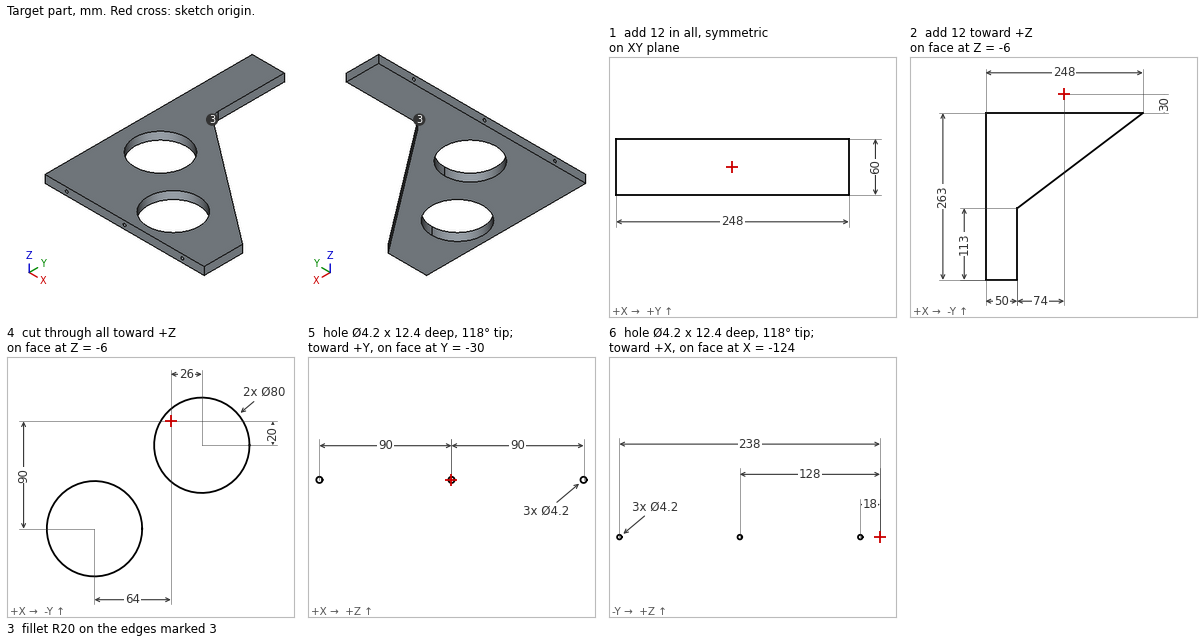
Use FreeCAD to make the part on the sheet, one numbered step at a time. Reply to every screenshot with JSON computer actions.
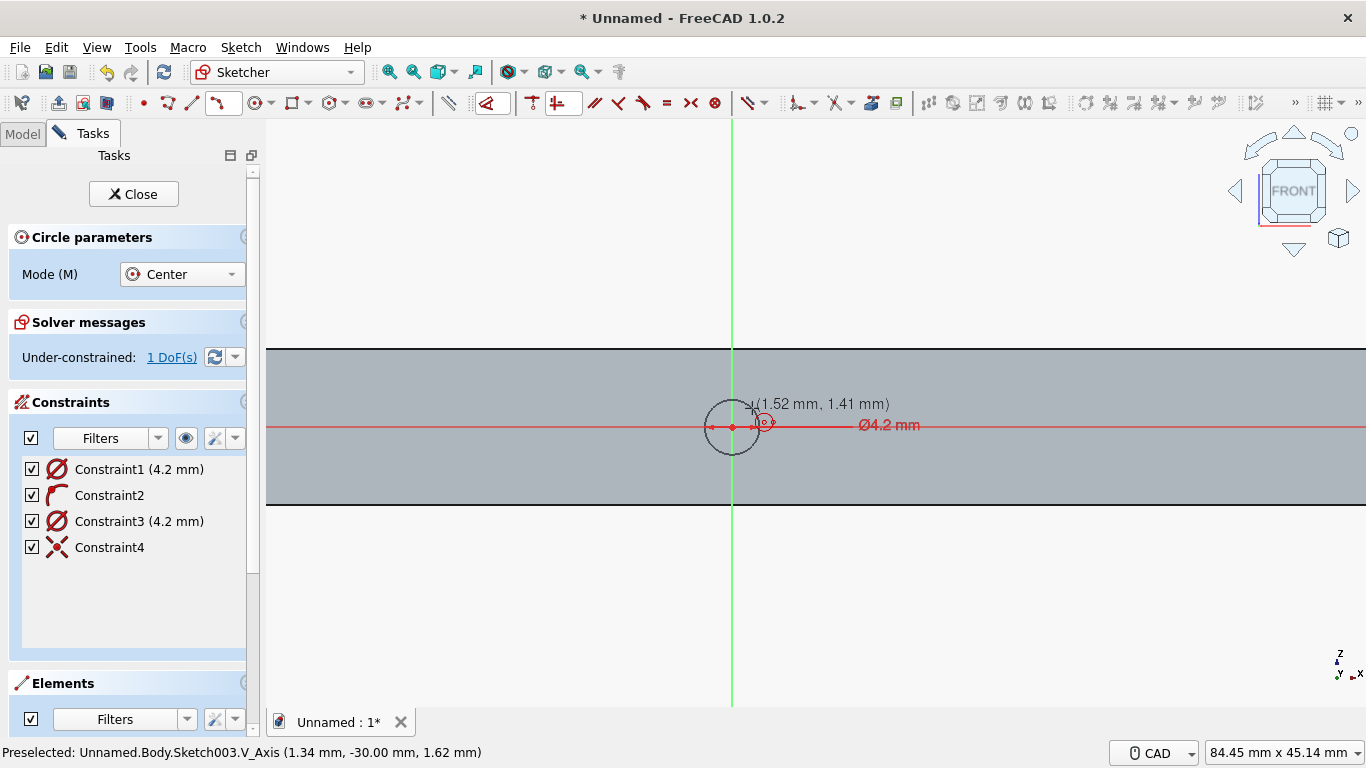
{"action": "scroll", "coordinate": [753, 408], "scroll_direction": "down", "scroll_amount": 7}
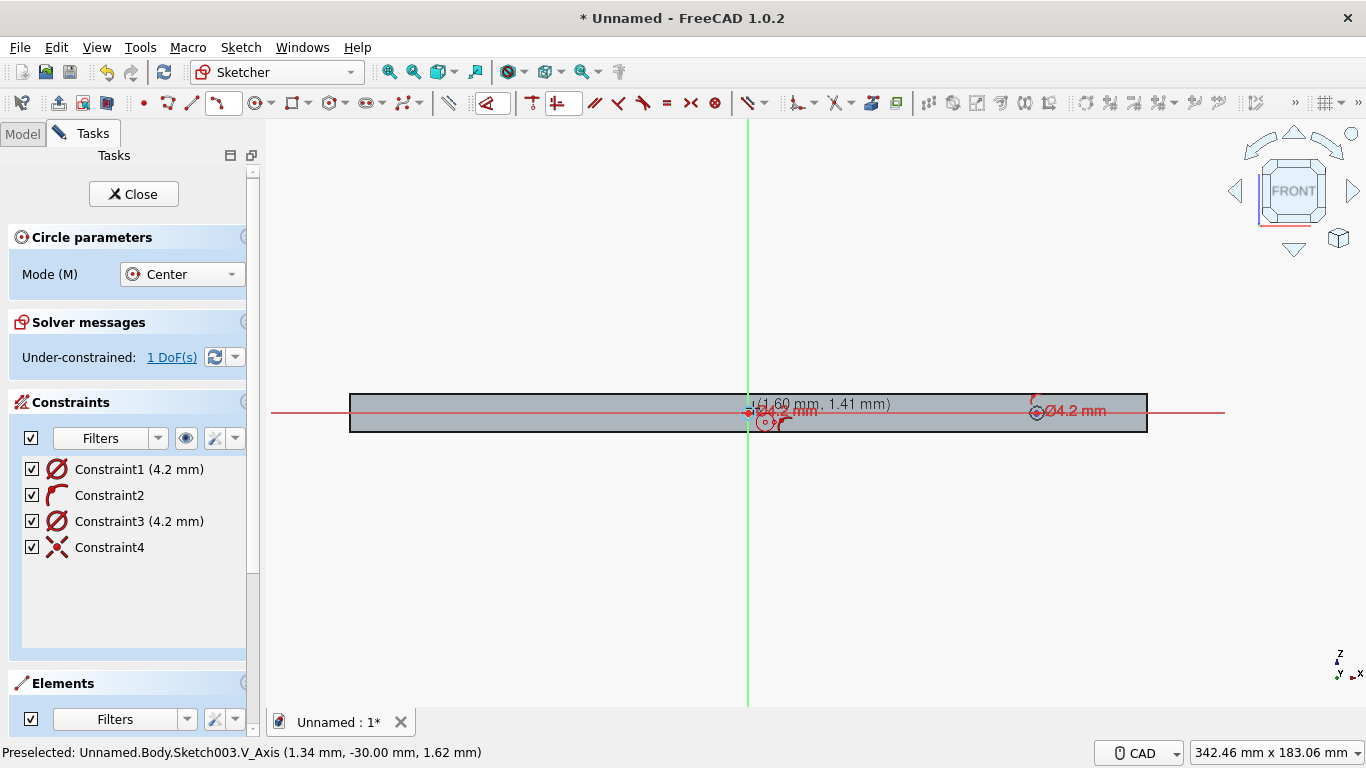
{"action": "scroll", "coordinate": [459, 413], "scroll_direction": "up", "scroll_amount": 7}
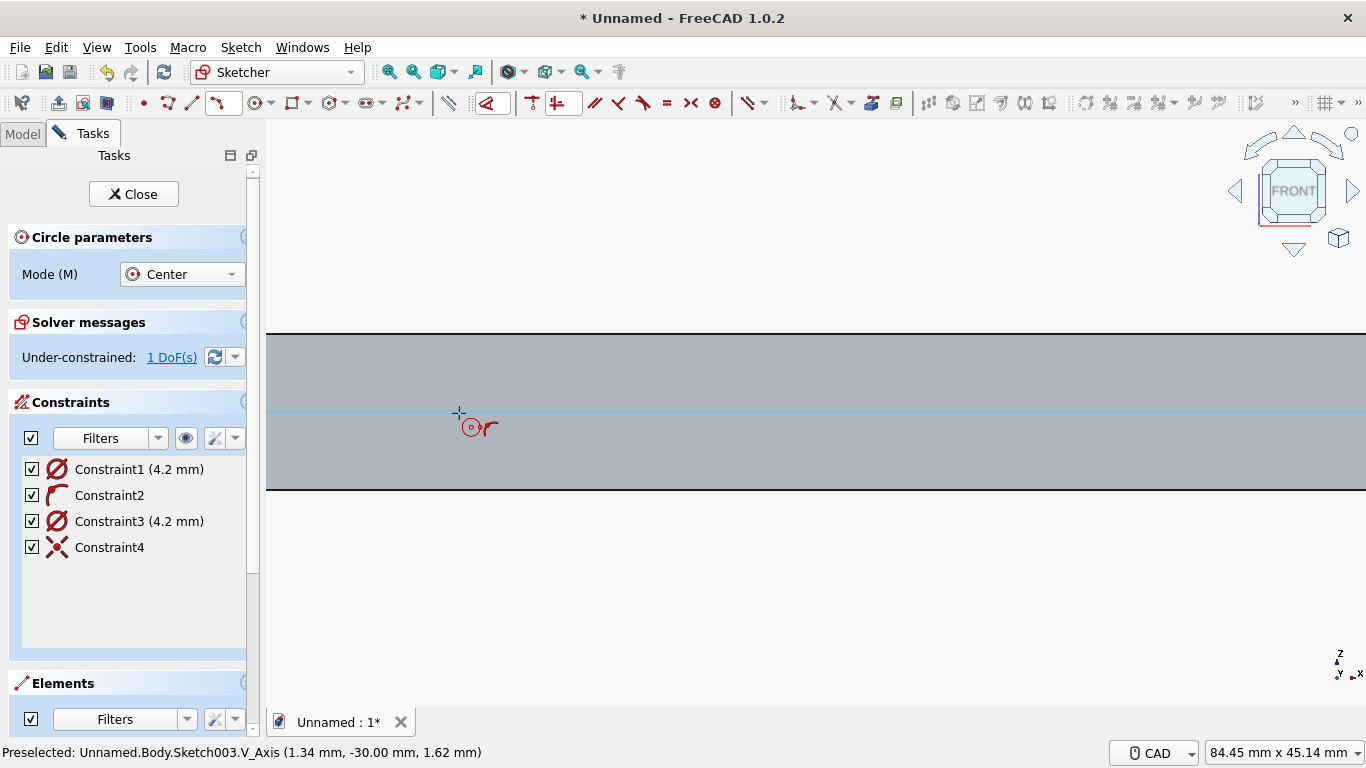
{"action": "scroll", "coordinate": [458, 413], "scroll_direction": "down", "scroll_amount": 7}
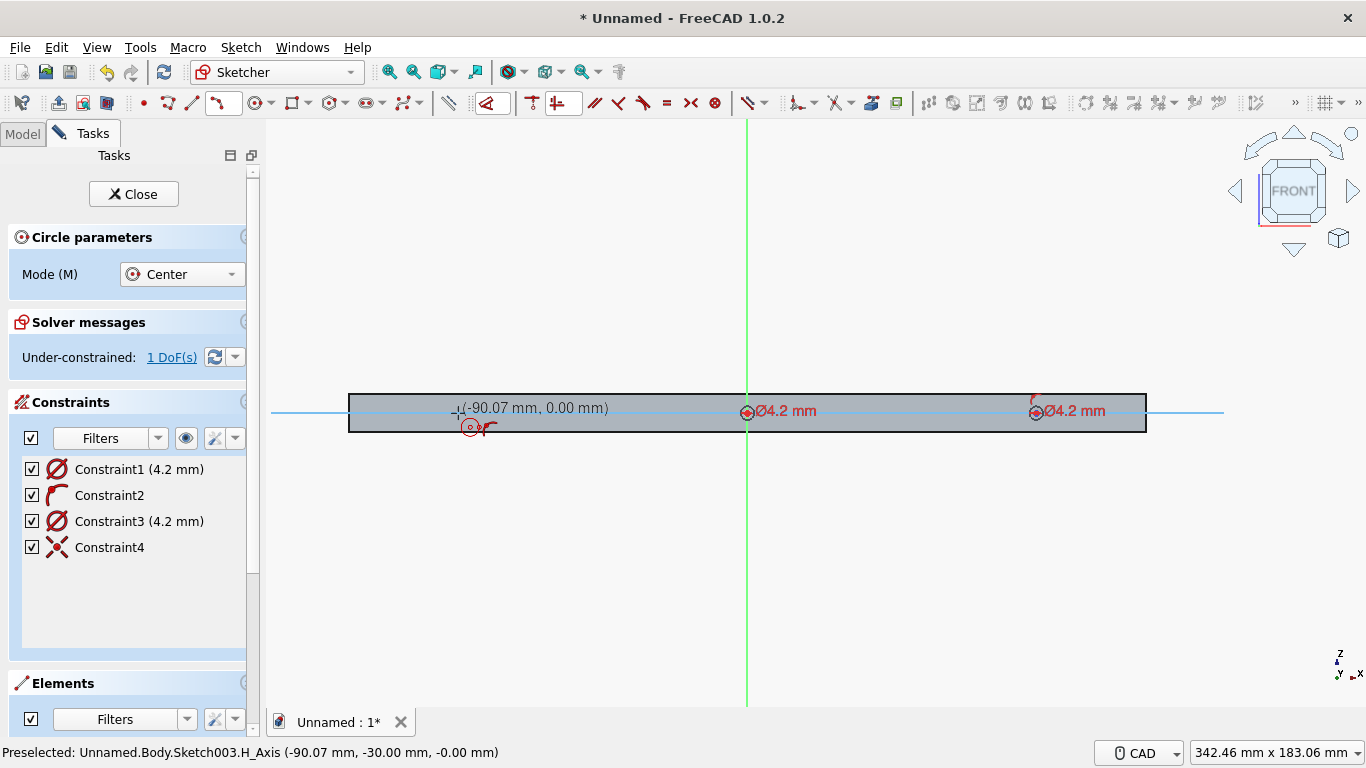
{"action": "left_click", "coordinate": [458, 413]}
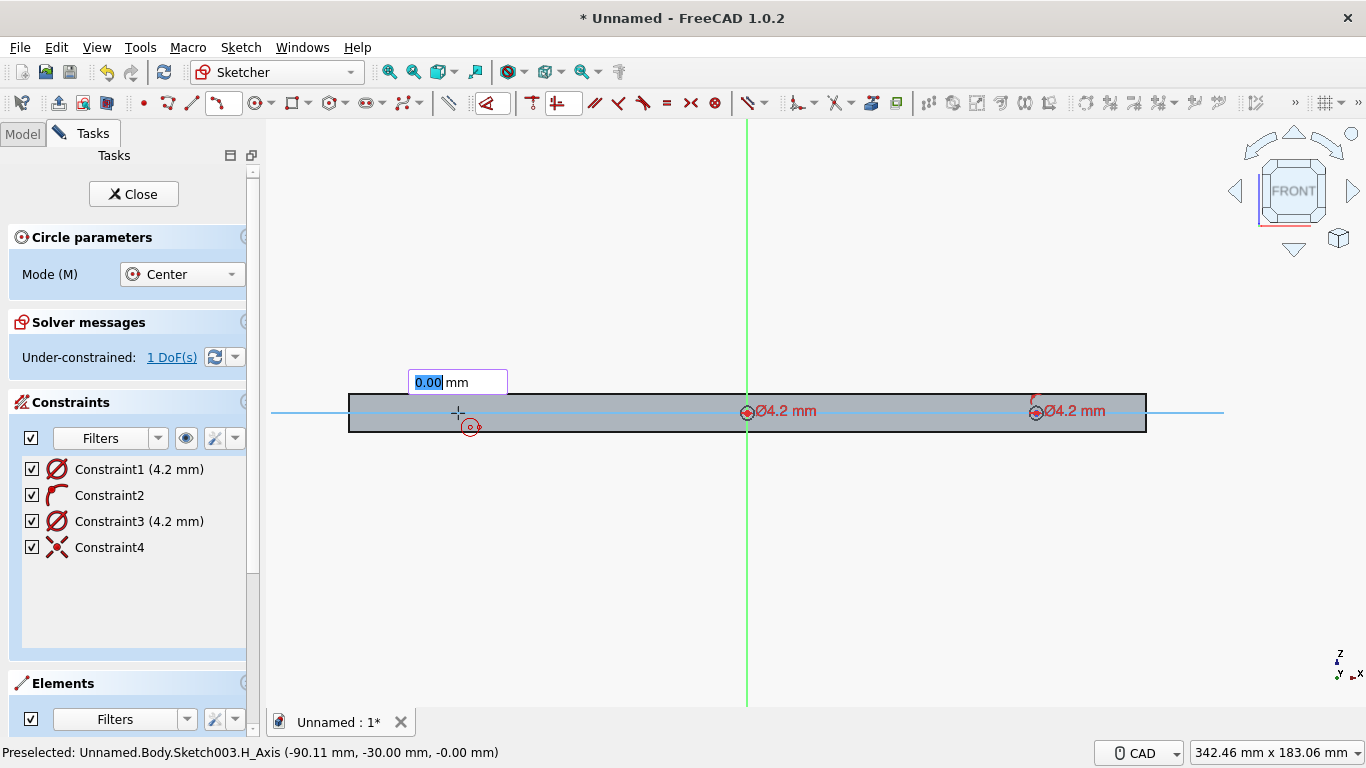
{"action": "scroll", "coordinate": [456, 419], "scroll_direction": "up", "scroll_amount": 5}
{"action": "mouse_move", "coordinate": [456, 419]}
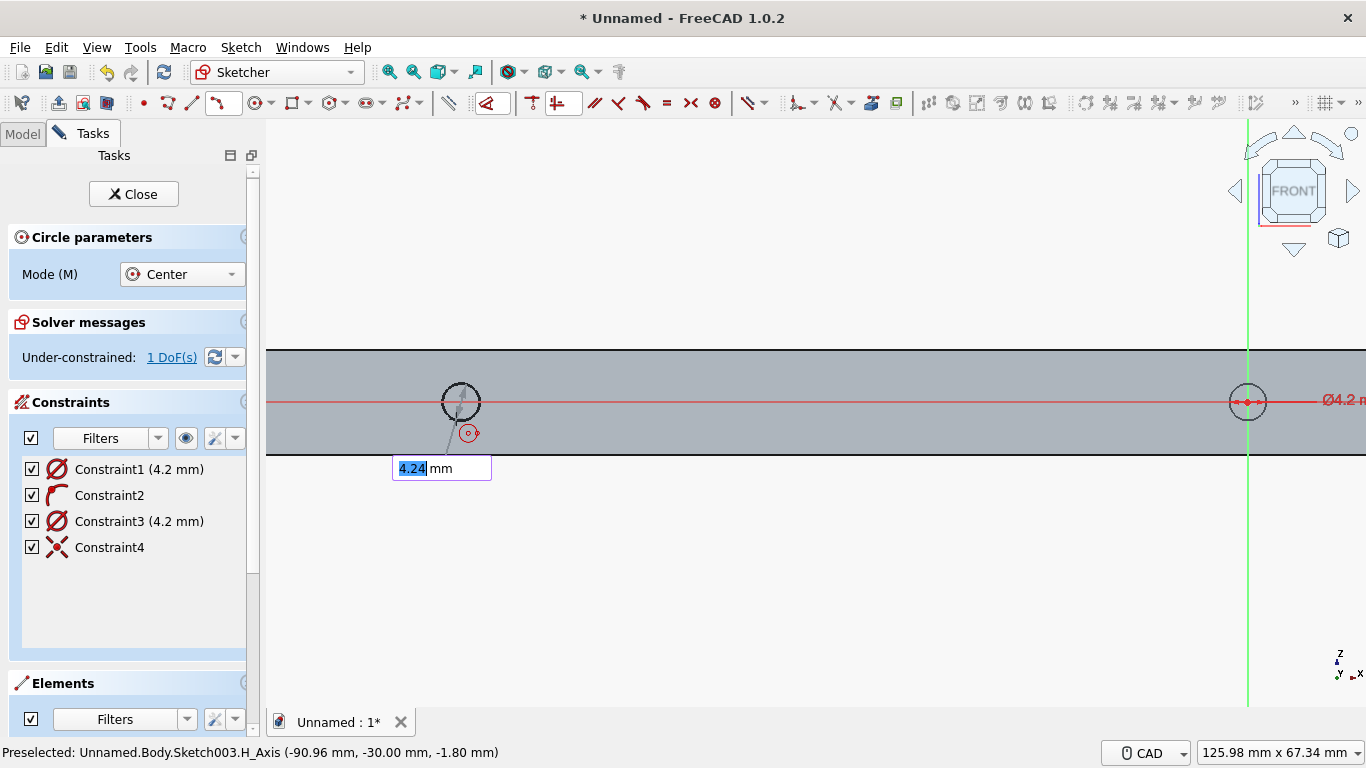
{"action": "type", "text": "4.2"}
{"action": "key", "text": "Return"}
{"action": "key", "text": "Escape"}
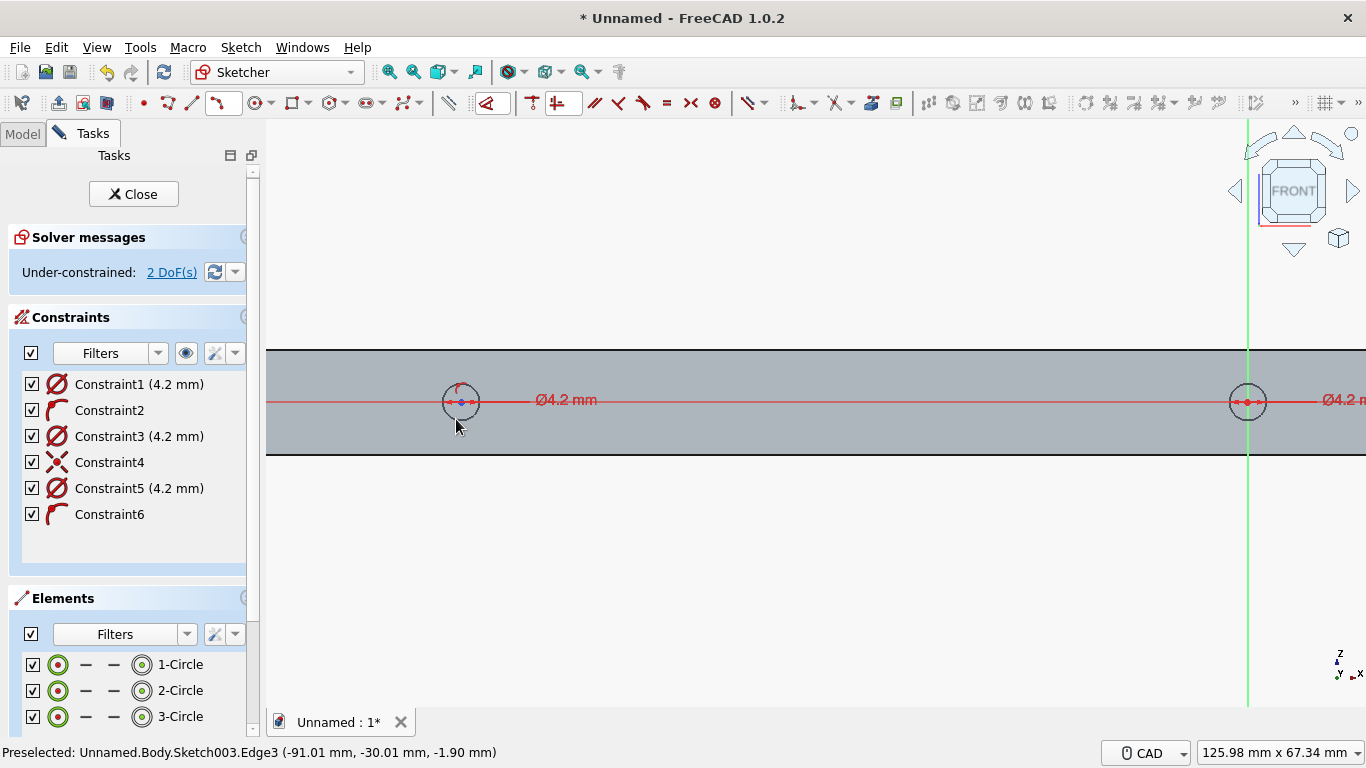
{"action": "scroll", "coordinate": [456, 419], "scroll_direction": "down", "scroll_amount": 5}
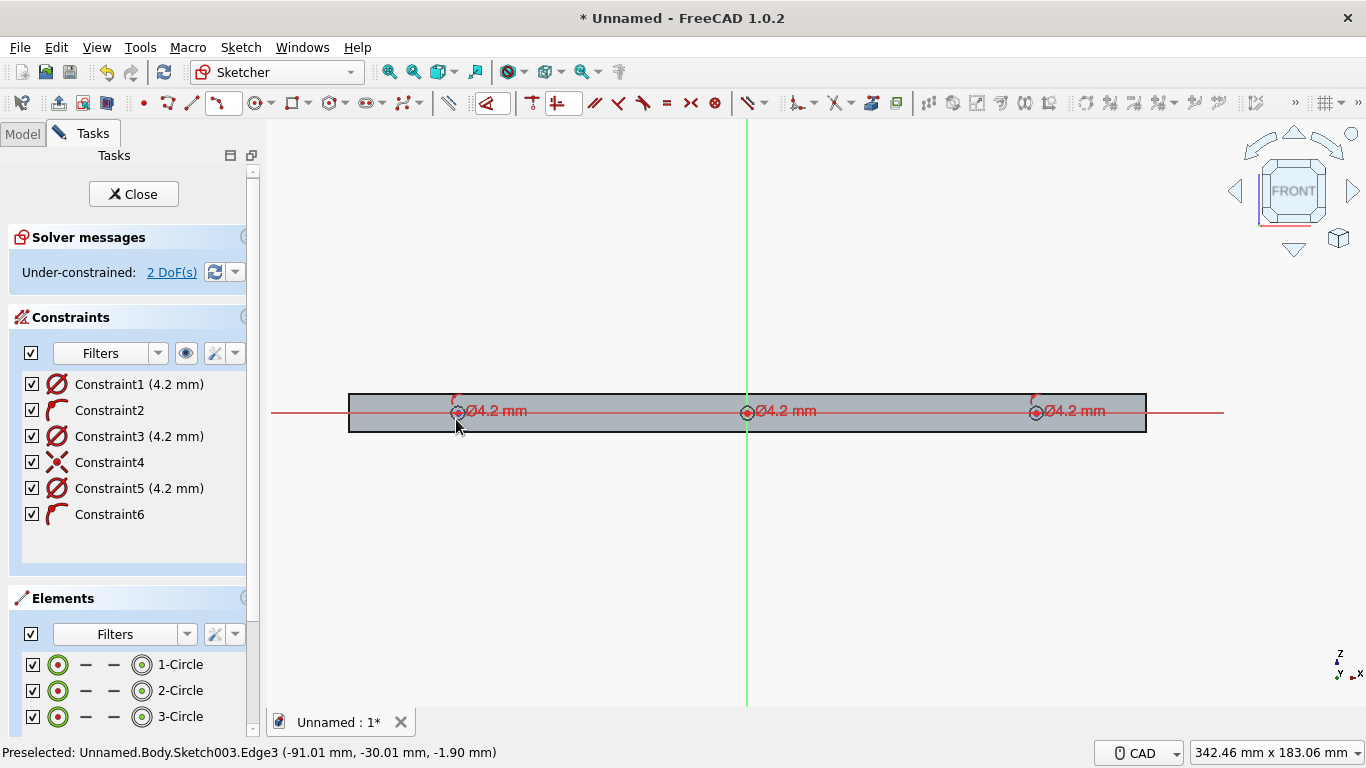
{"action": "left_click", "coordinate": [1036, 413]}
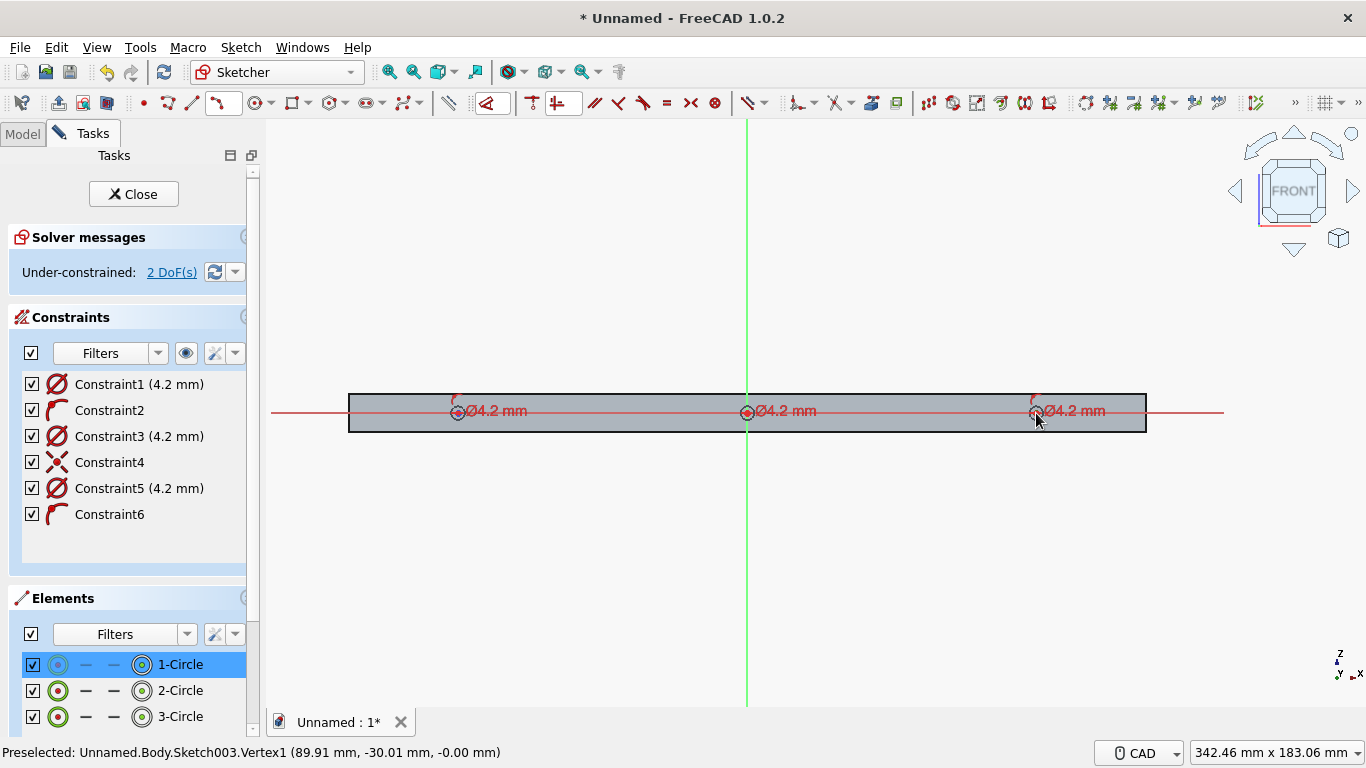
{"action": "key", "text": "l"}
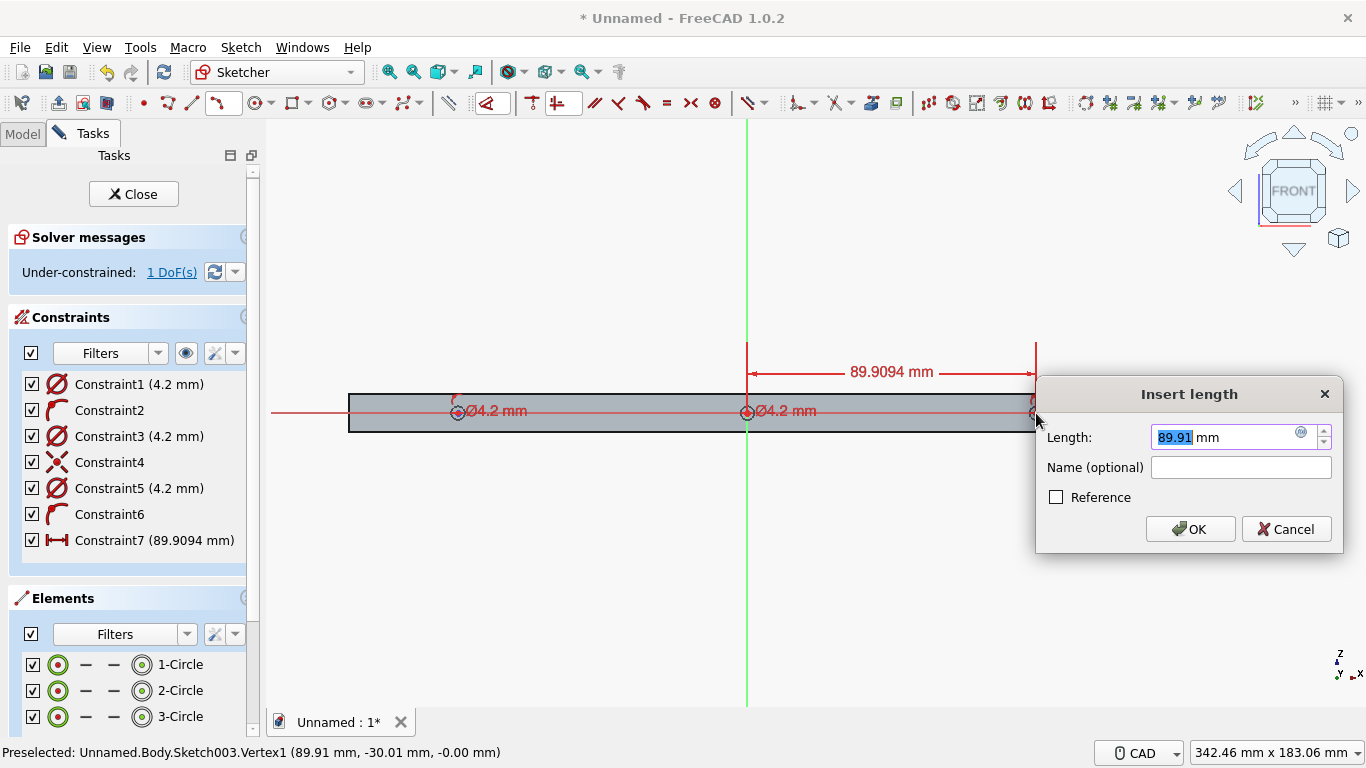
{"action": "type", "text": "90"}
{"action": "key", "text": "Return"}